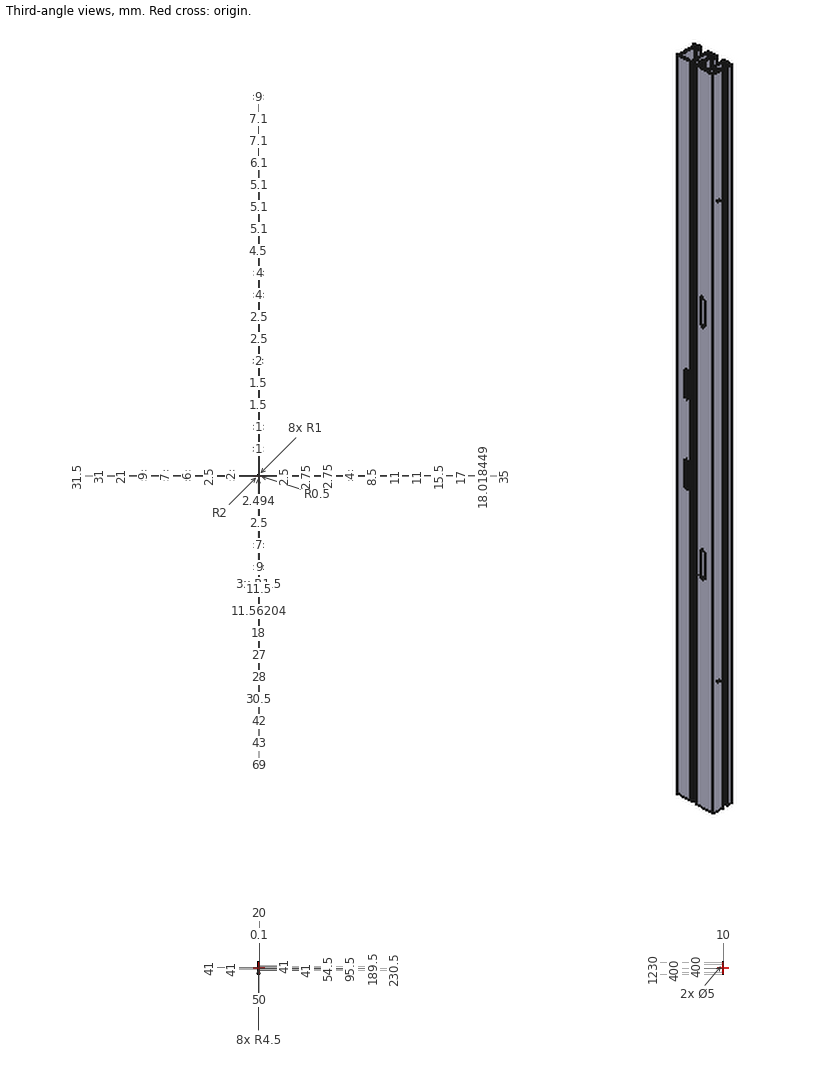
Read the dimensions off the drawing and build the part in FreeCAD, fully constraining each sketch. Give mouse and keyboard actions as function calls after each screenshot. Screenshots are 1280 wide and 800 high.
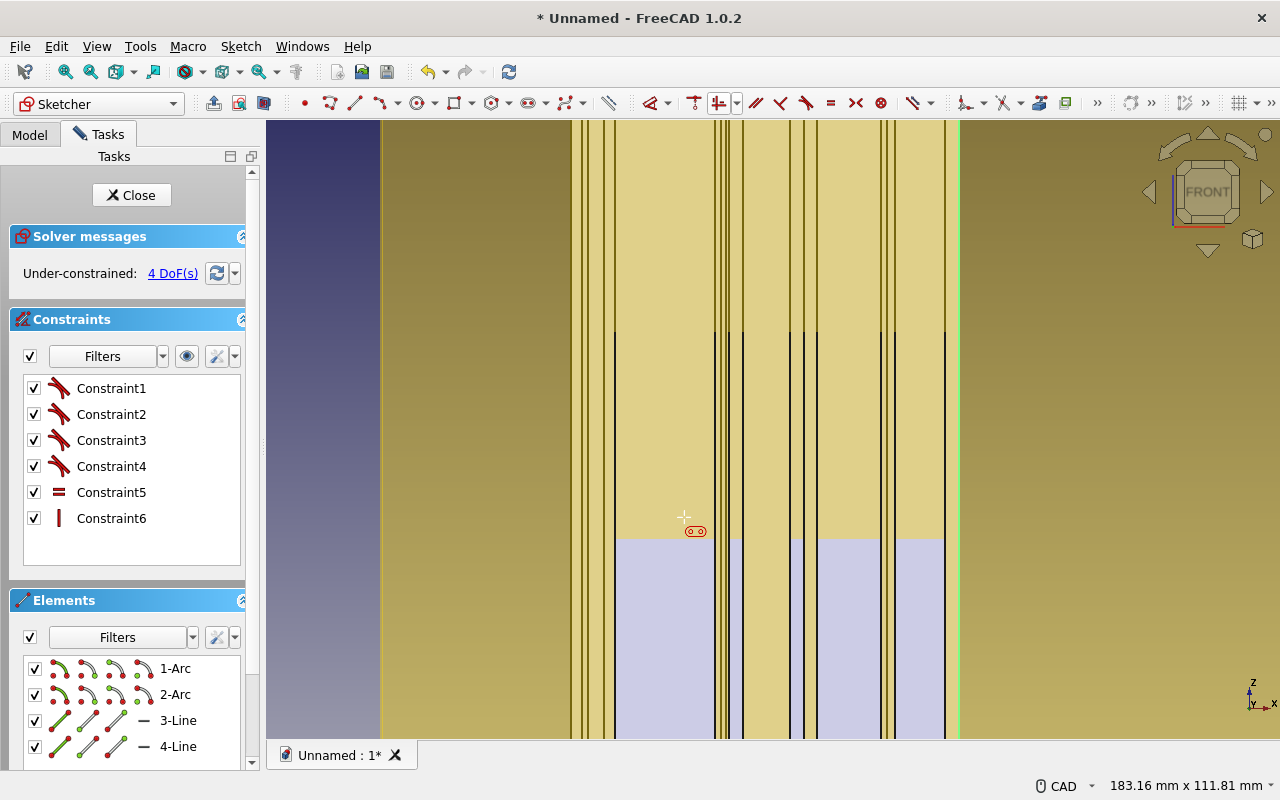
scroll(684, 518, down, 9)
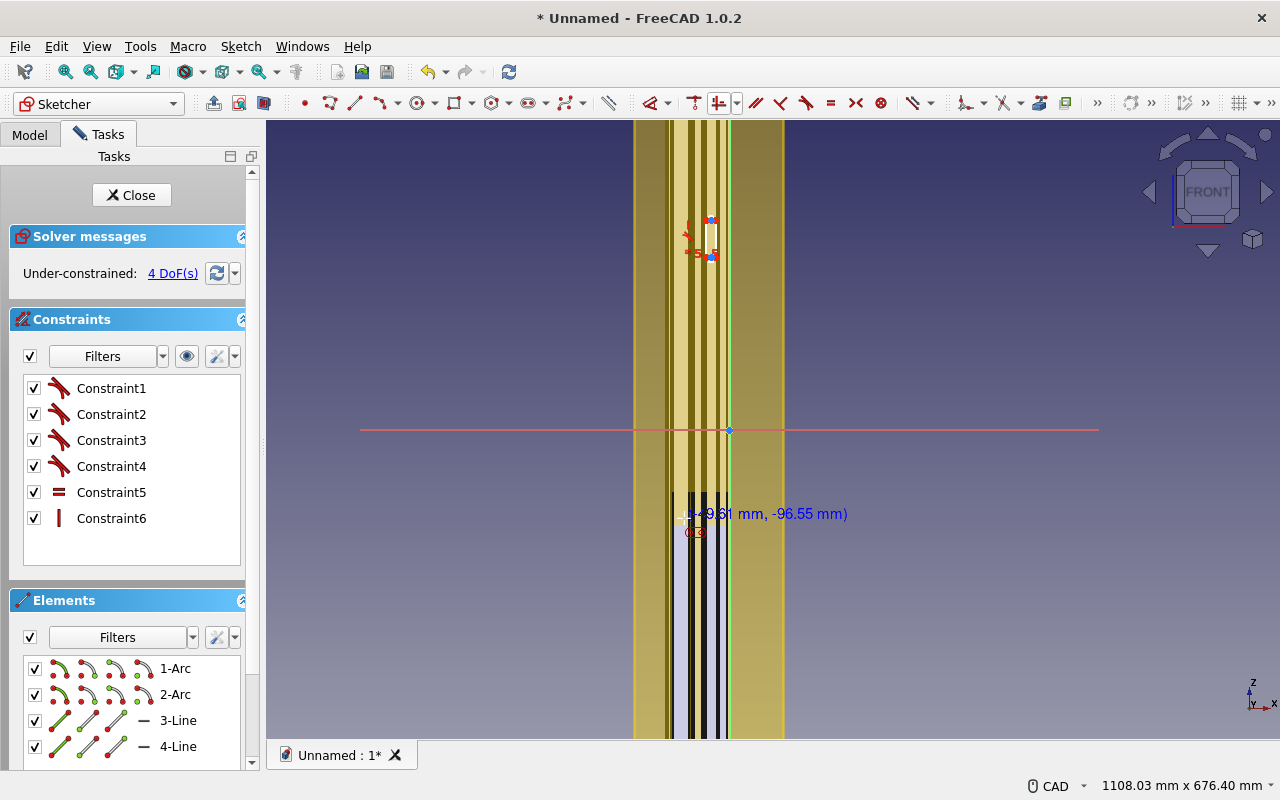
click(684, 518)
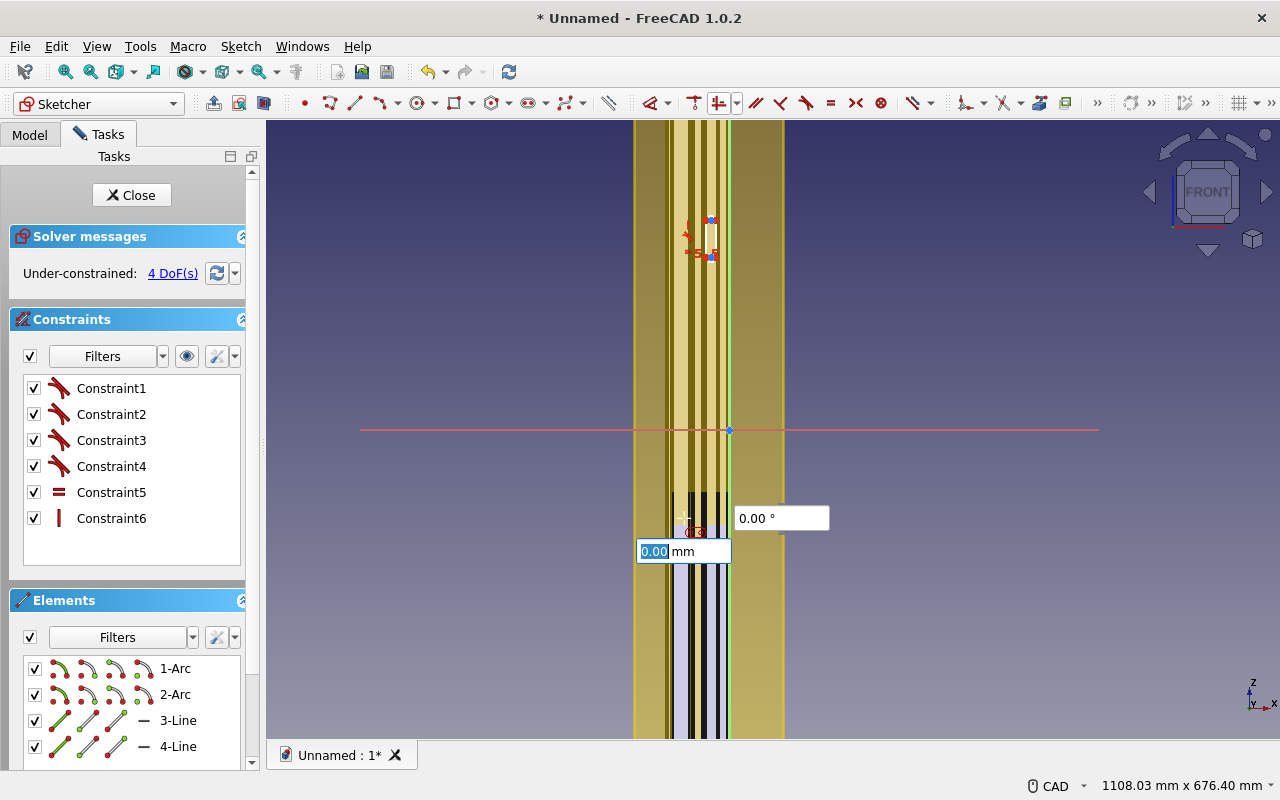
click(684, 480)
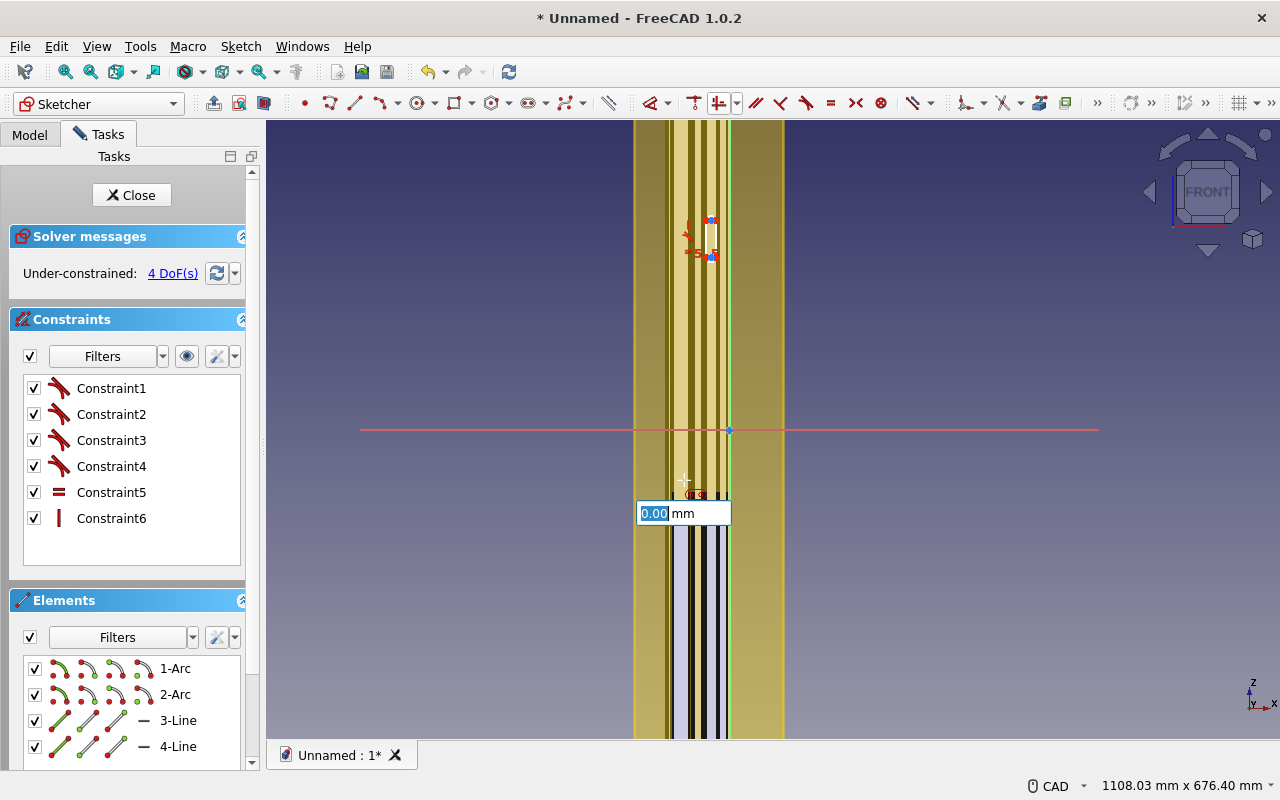
scroll(688, 499, up, 7)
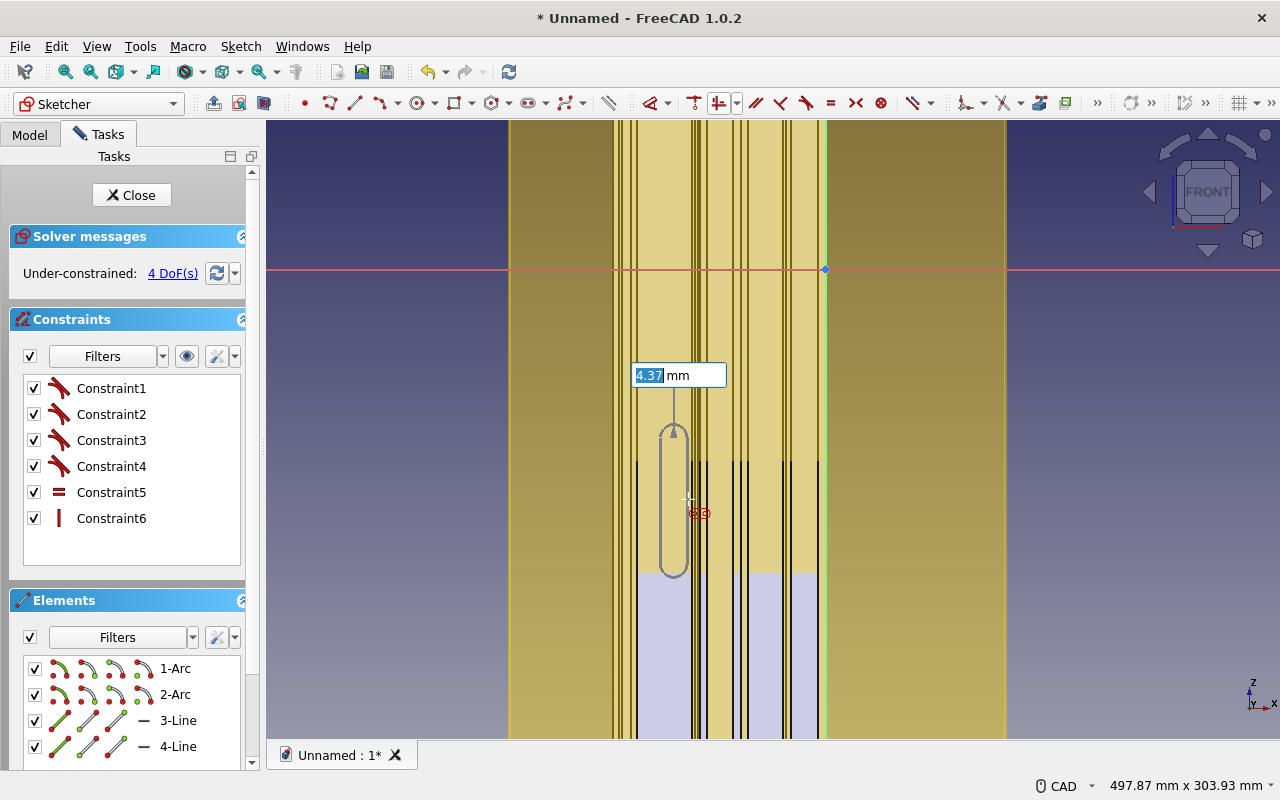
click(687, 497)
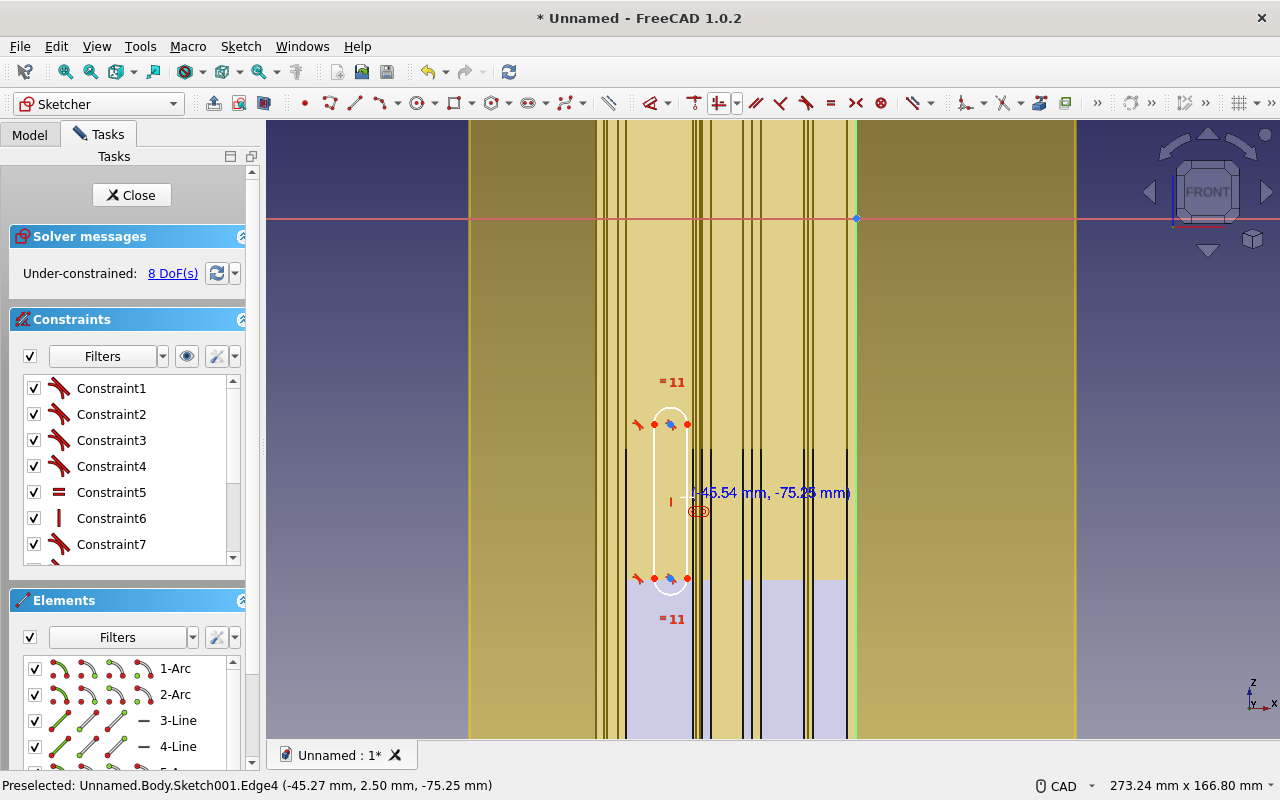
scroll(688, 498, down, 7)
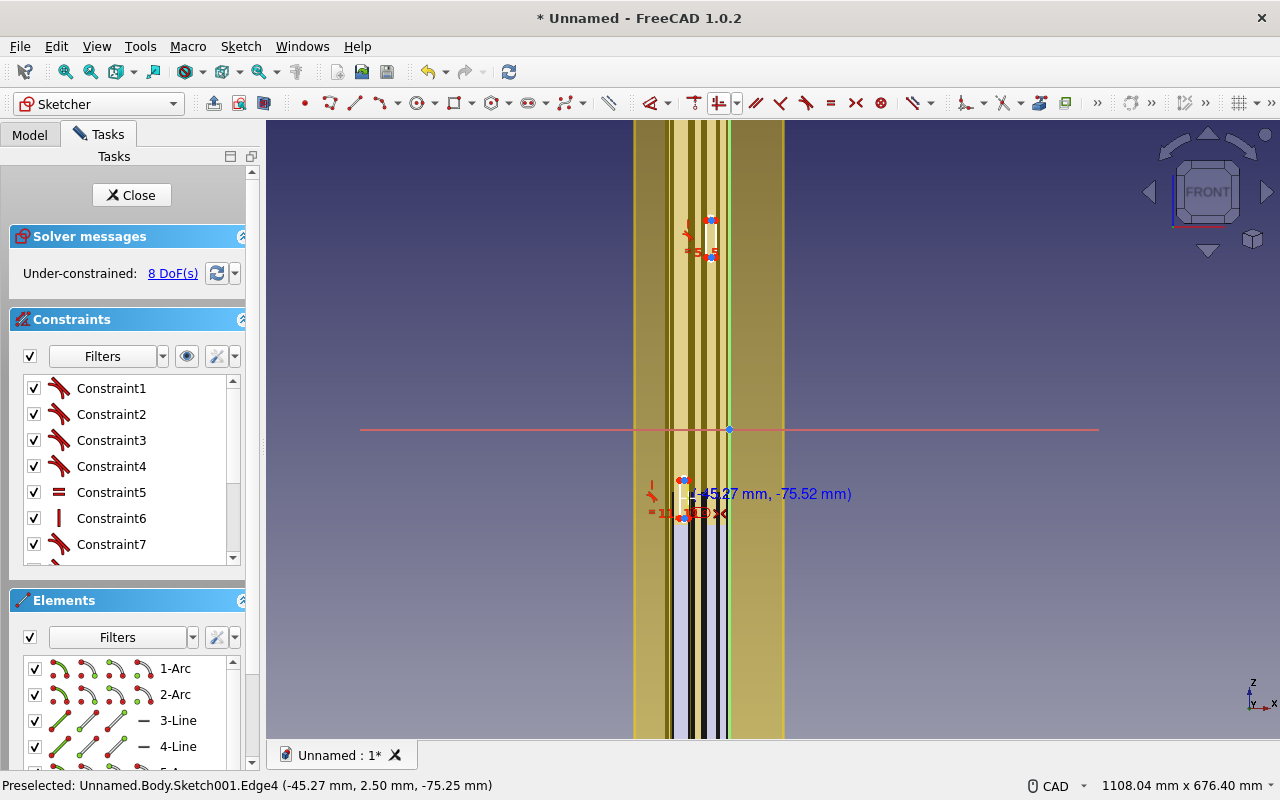
scroll(684, 380, up, 9)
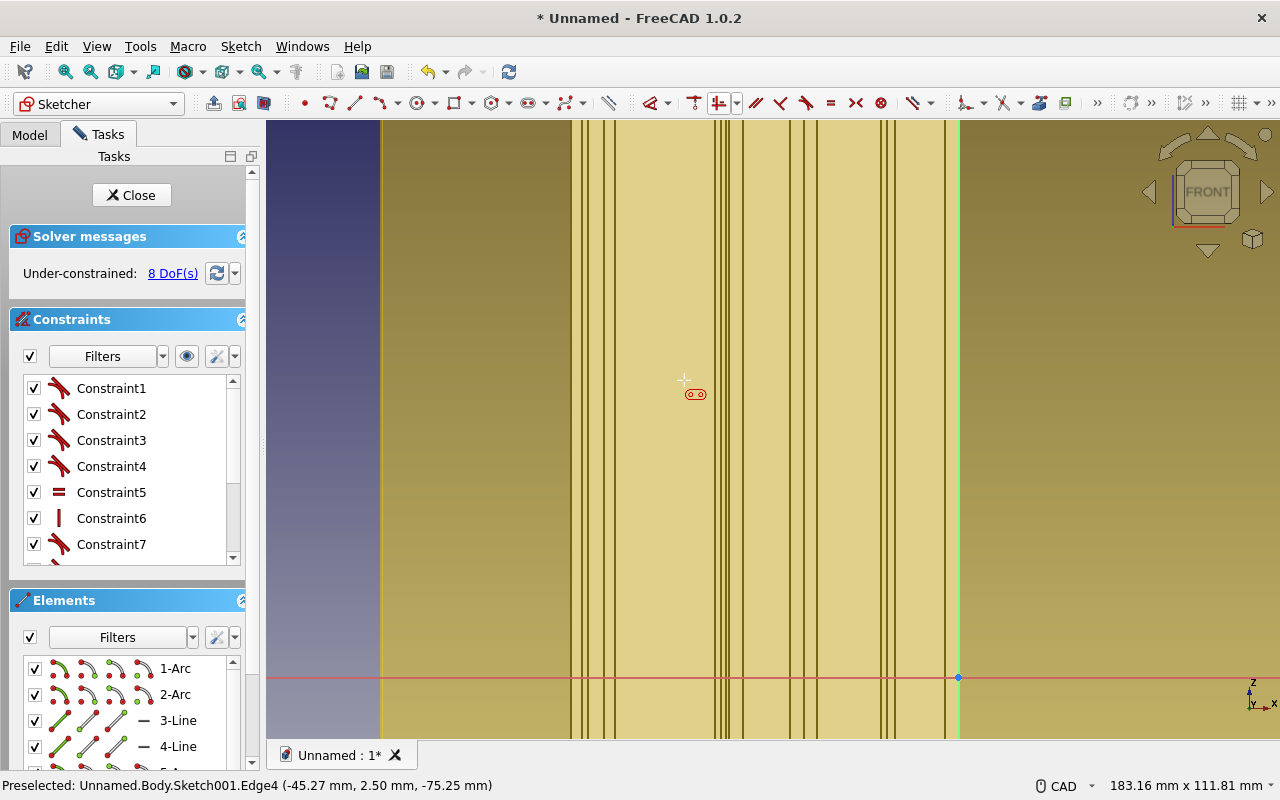
scroll(684, 380, down, 9)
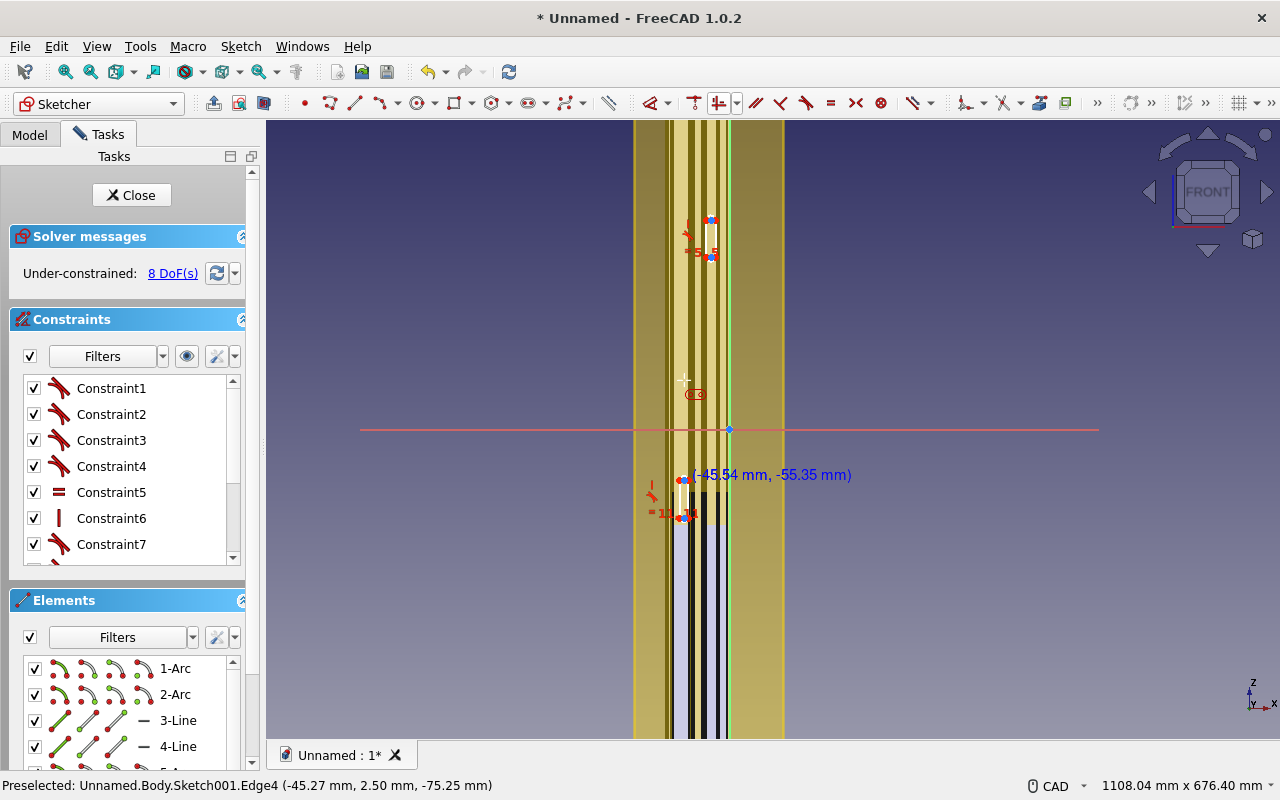
click(684, 380)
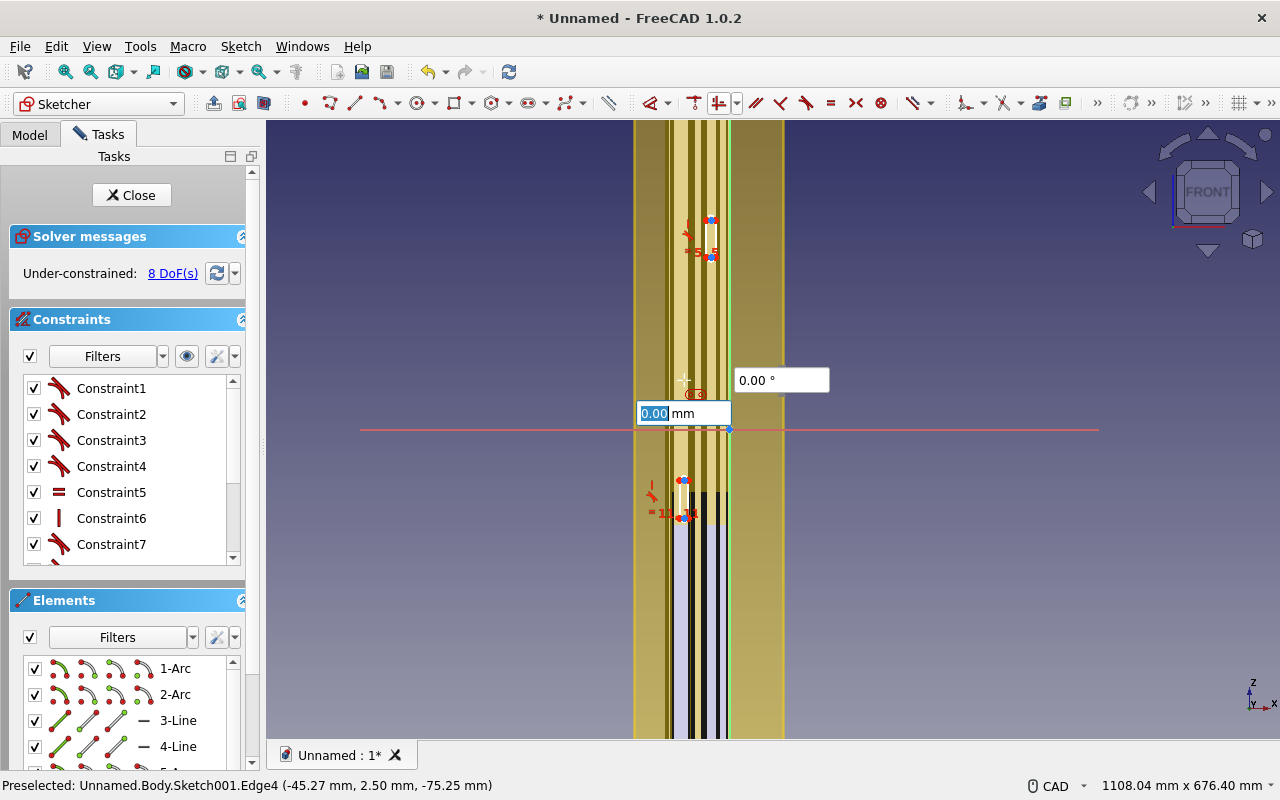
click(684, 342)